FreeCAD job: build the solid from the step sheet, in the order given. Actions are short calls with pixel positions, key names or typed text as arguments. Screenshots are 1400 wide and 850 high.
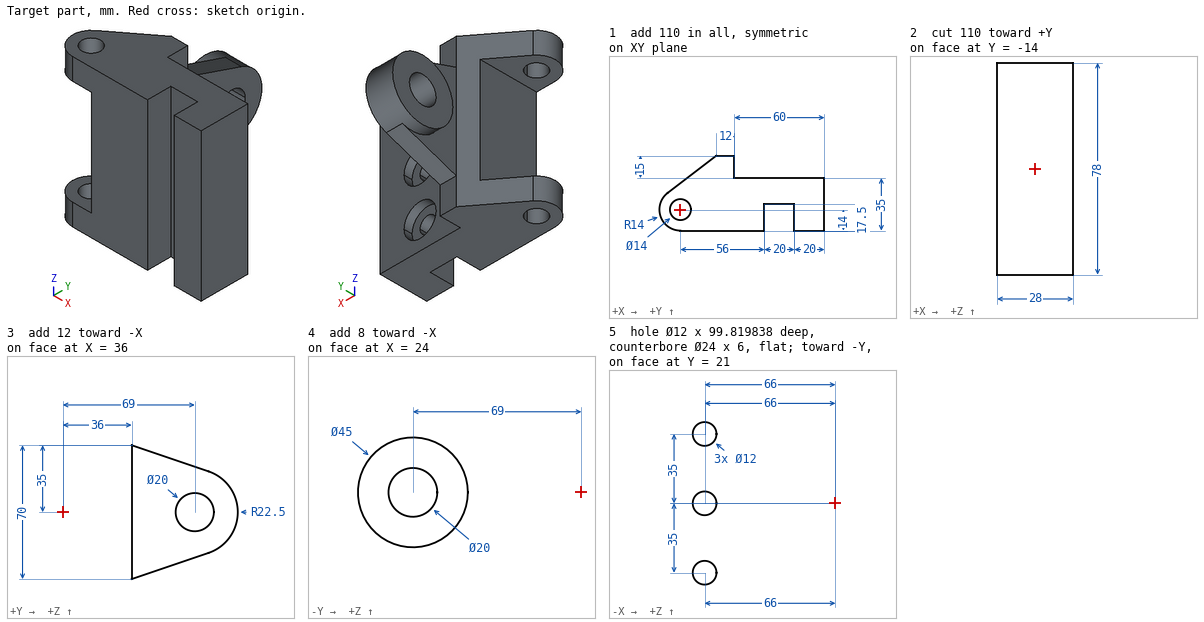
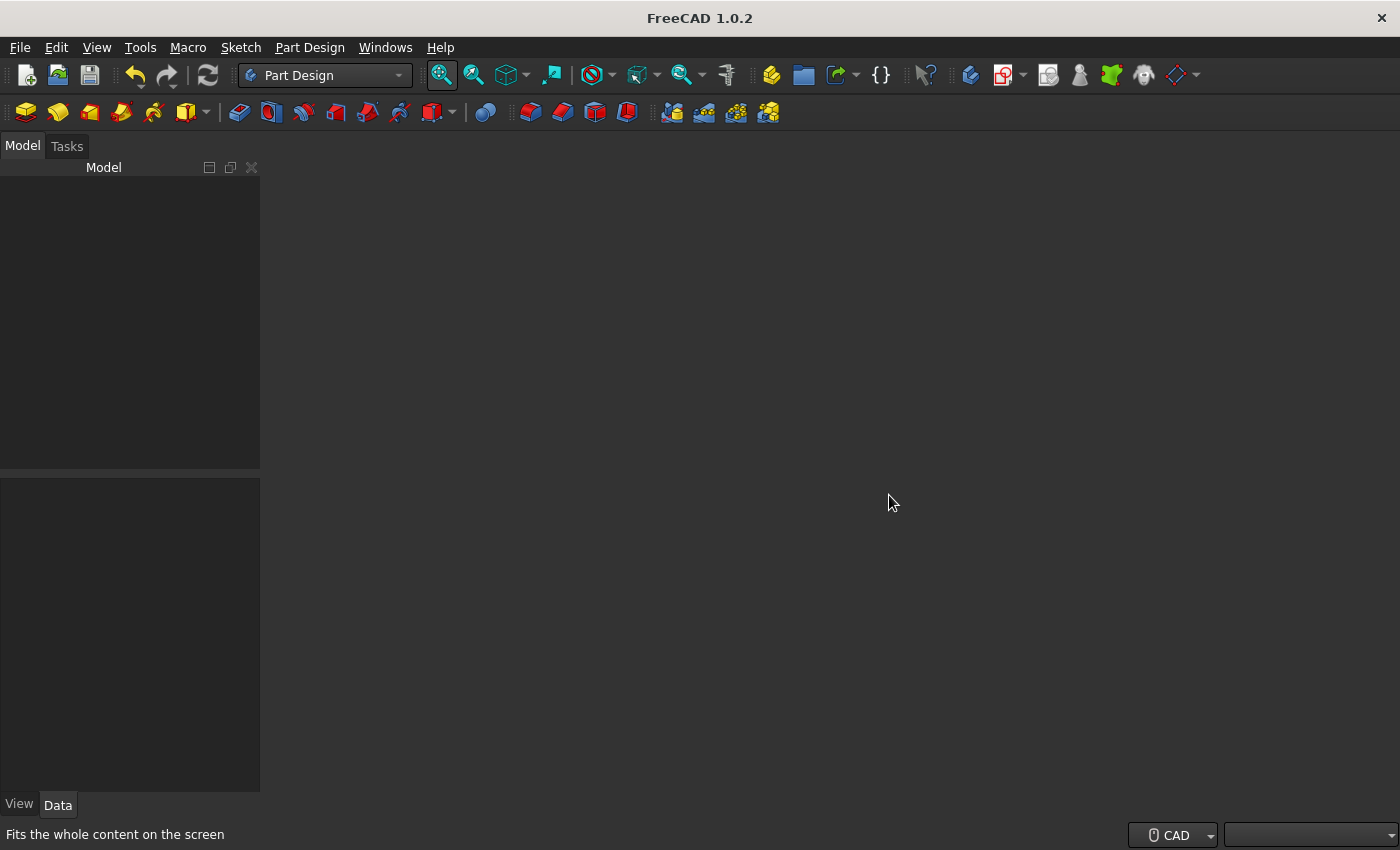
click(26, 76)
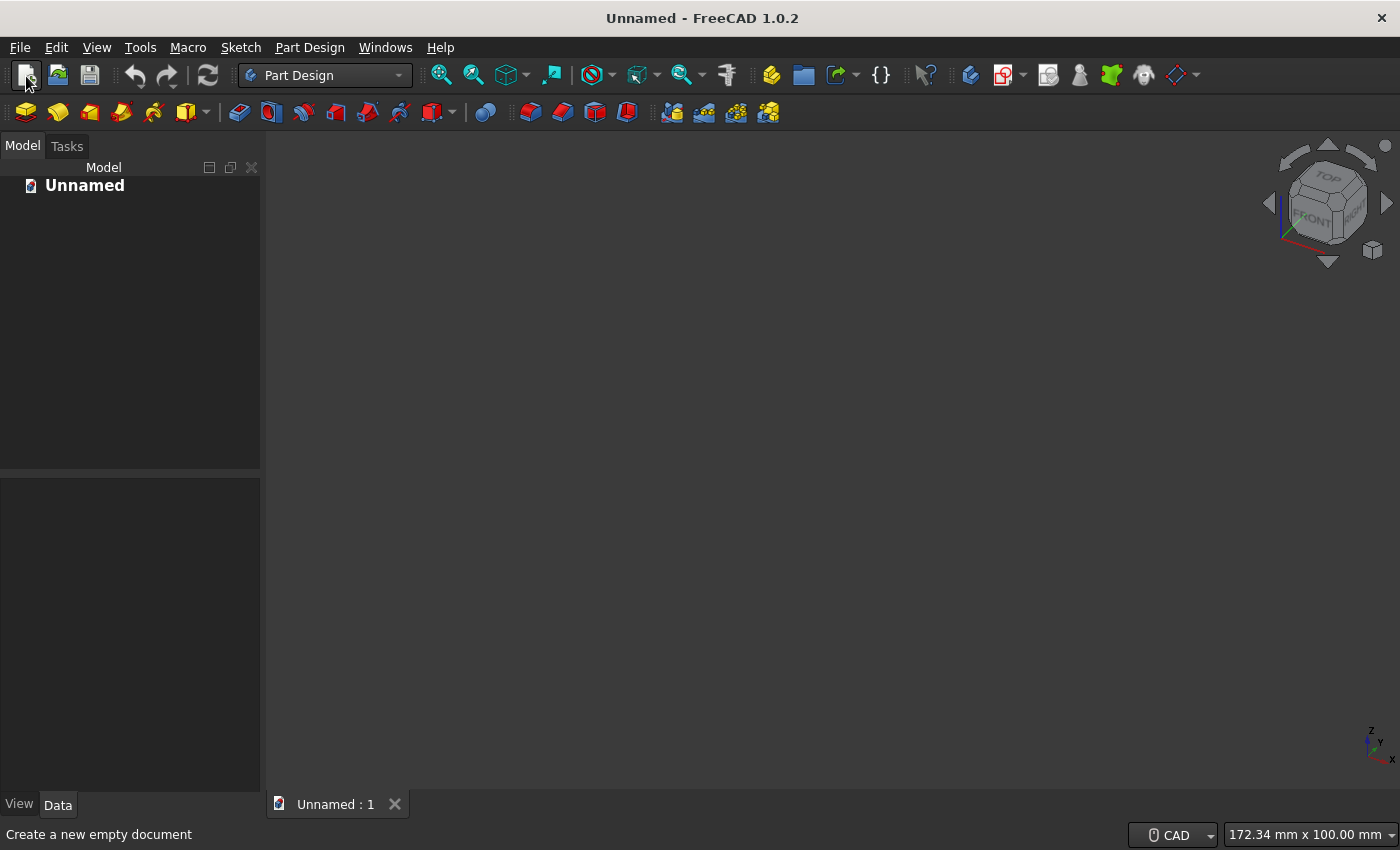
click(1004, 76)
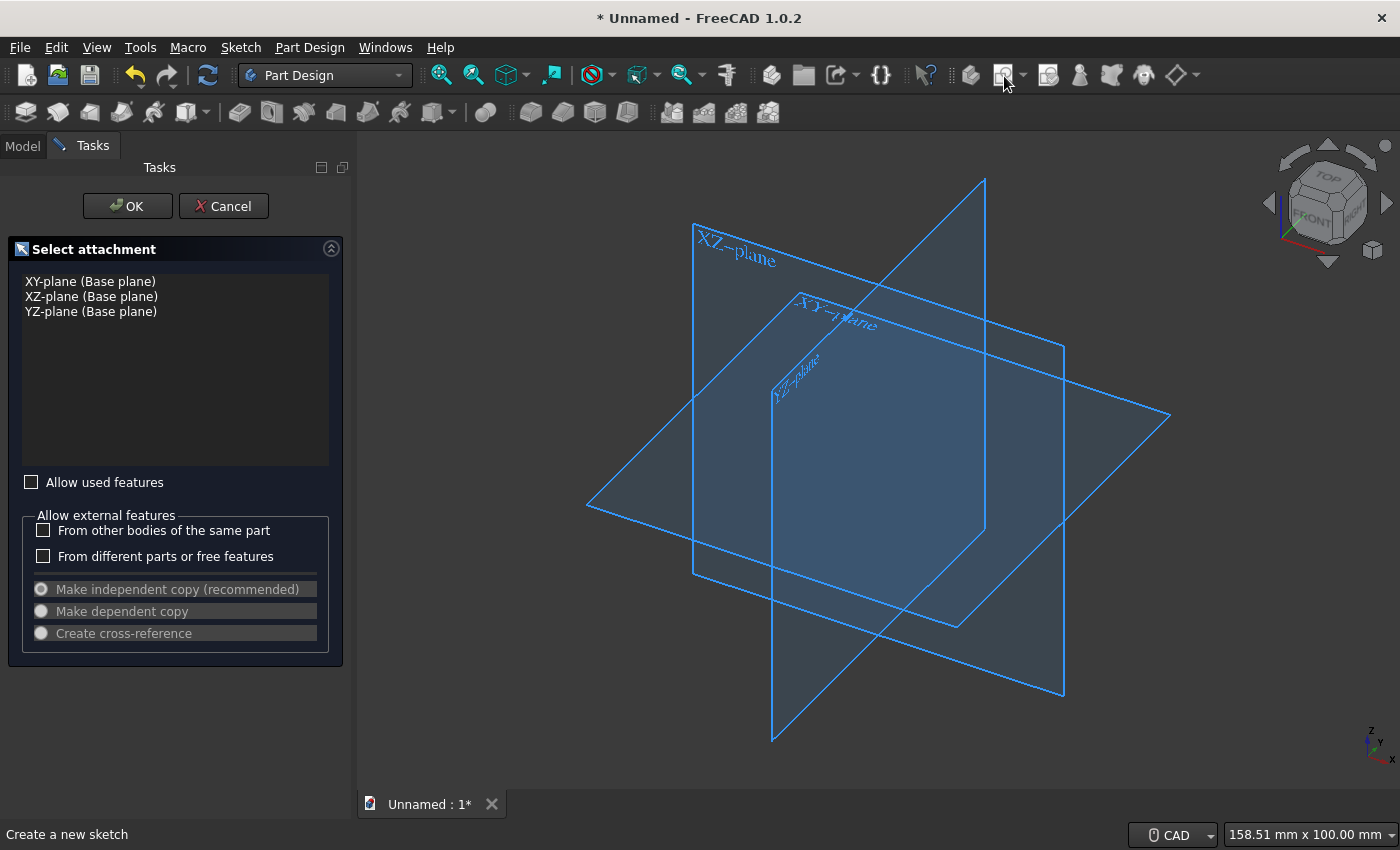
click(82, 282)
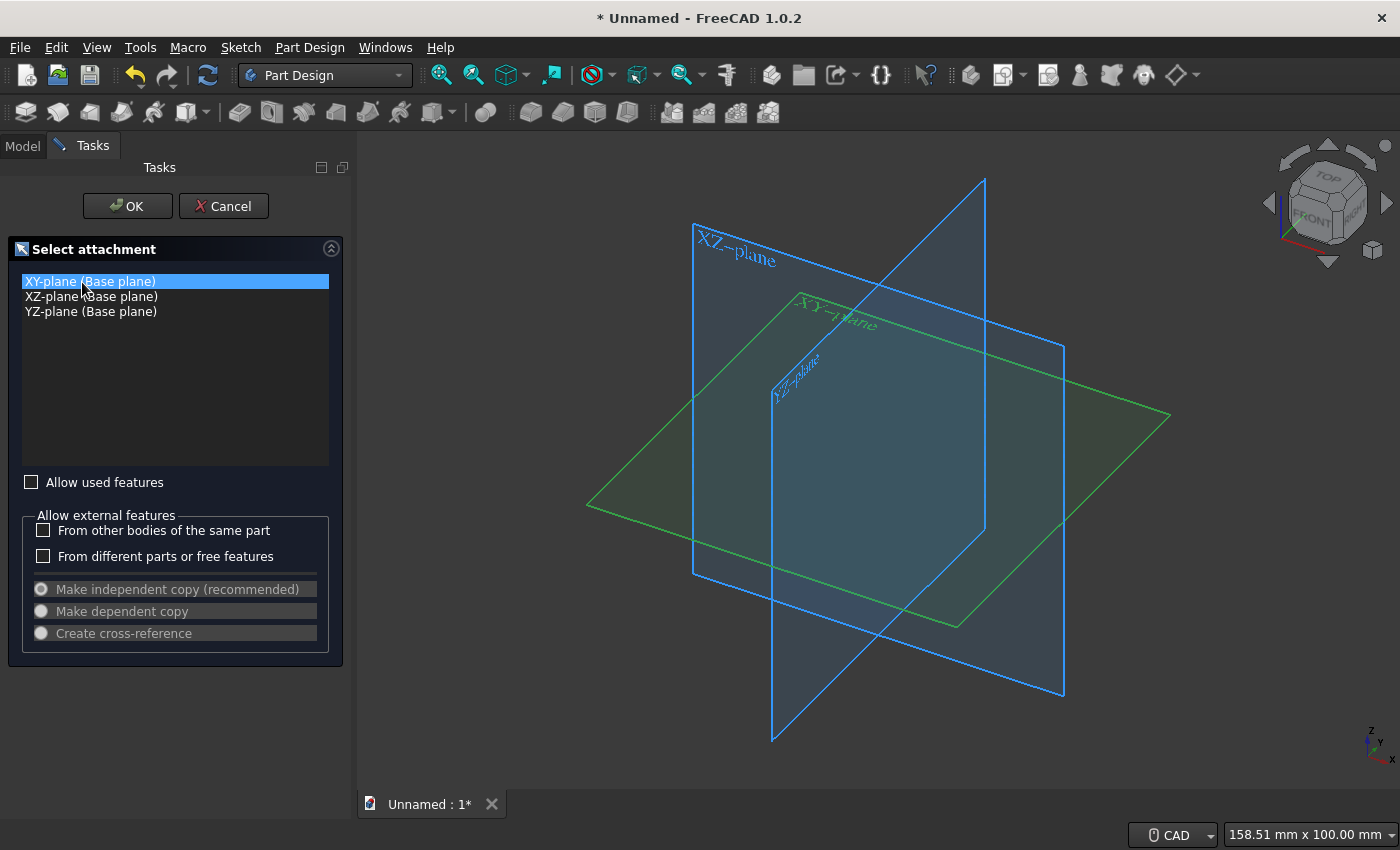
click(128, 206)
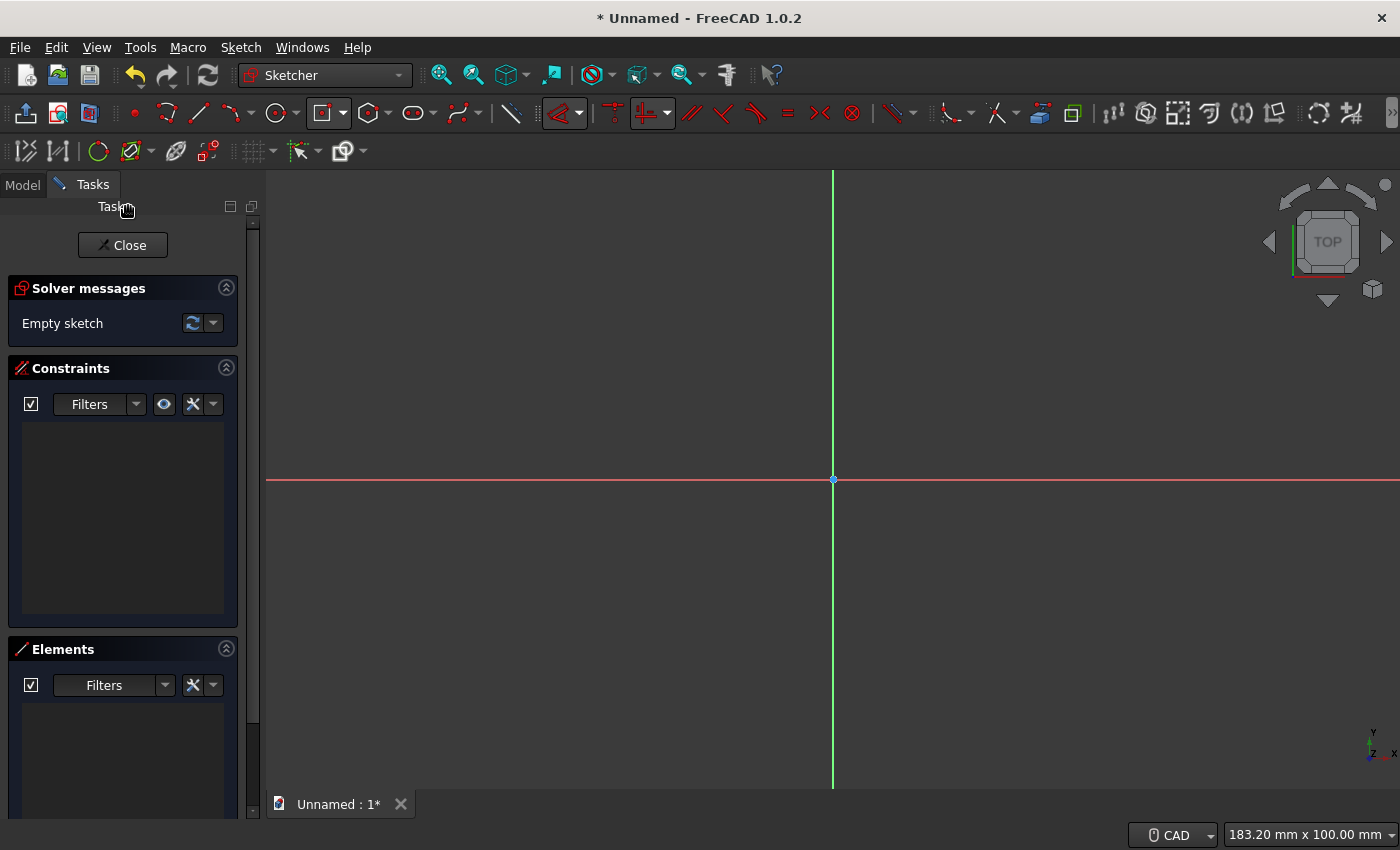
scroll(294, 618, down, 2)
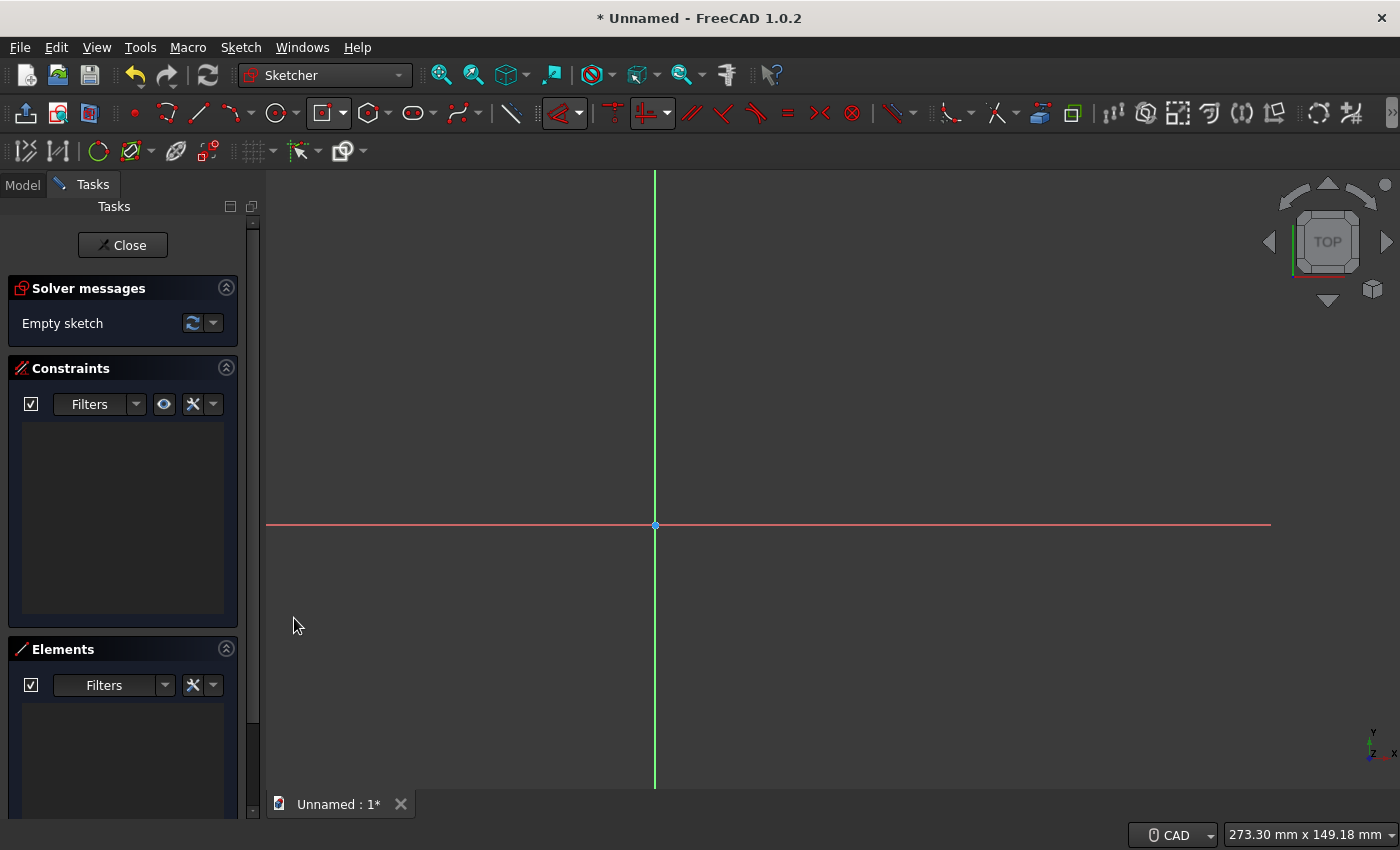
scroll(954, 480, up, 2)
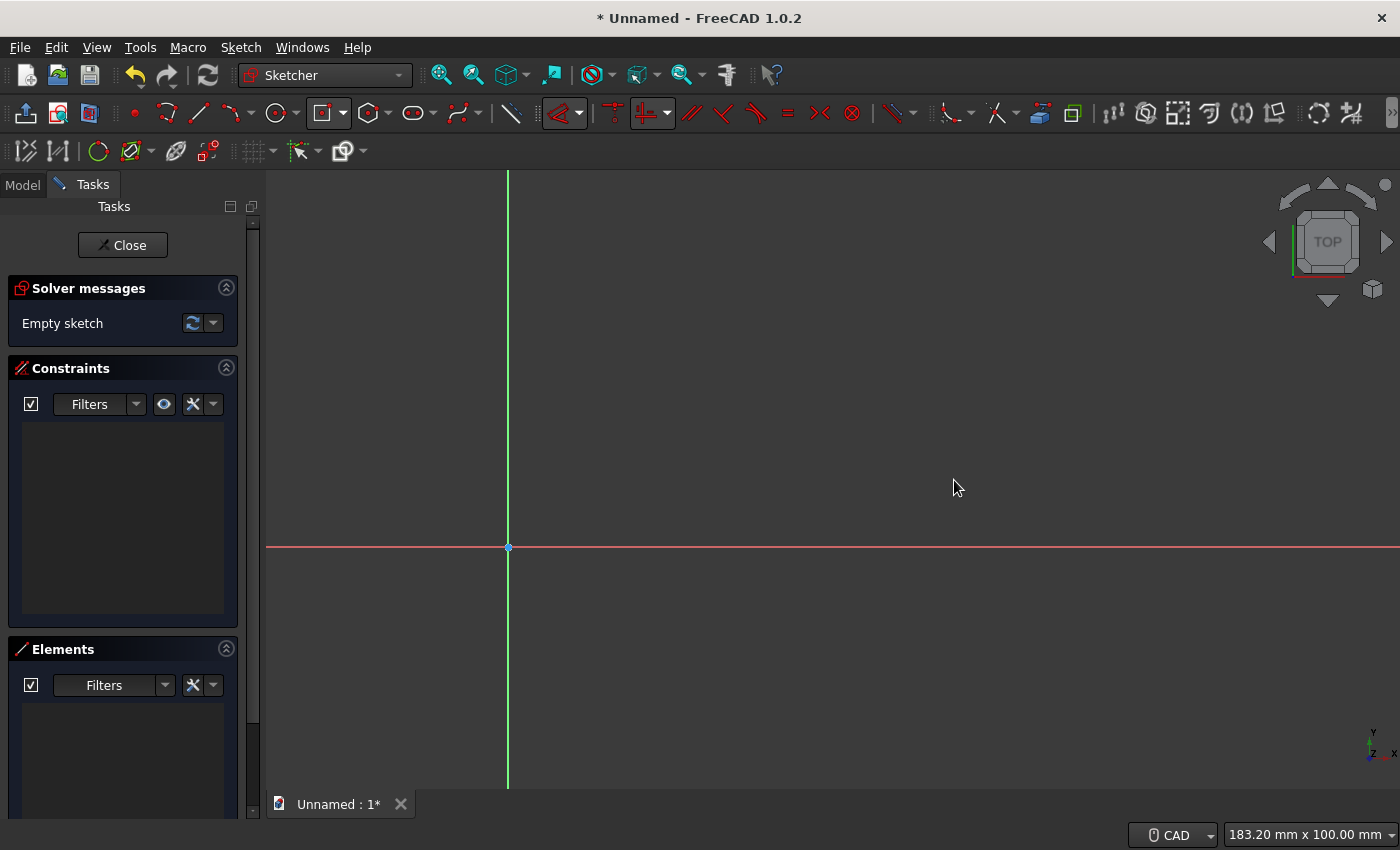
click(168, 114)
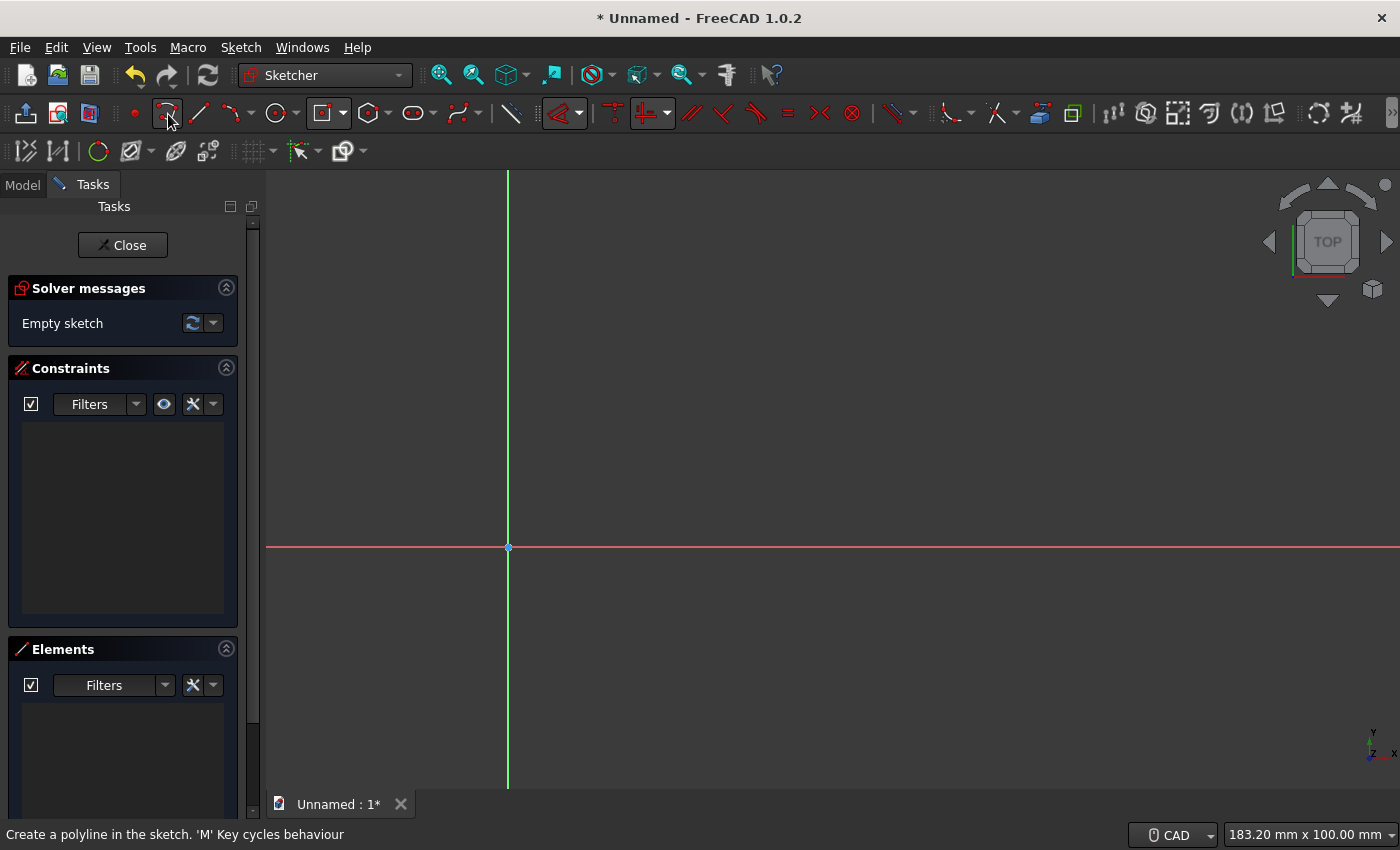
click(508, 634)
click(855, 634)
click(855, 526)
click(979, 526)
click(979, 634)
click(1102, 634)
click(1102, 417)
click(731, 417)
click(731, 325)
click(657, 325)
click(455, 479)
right_click(455, 479)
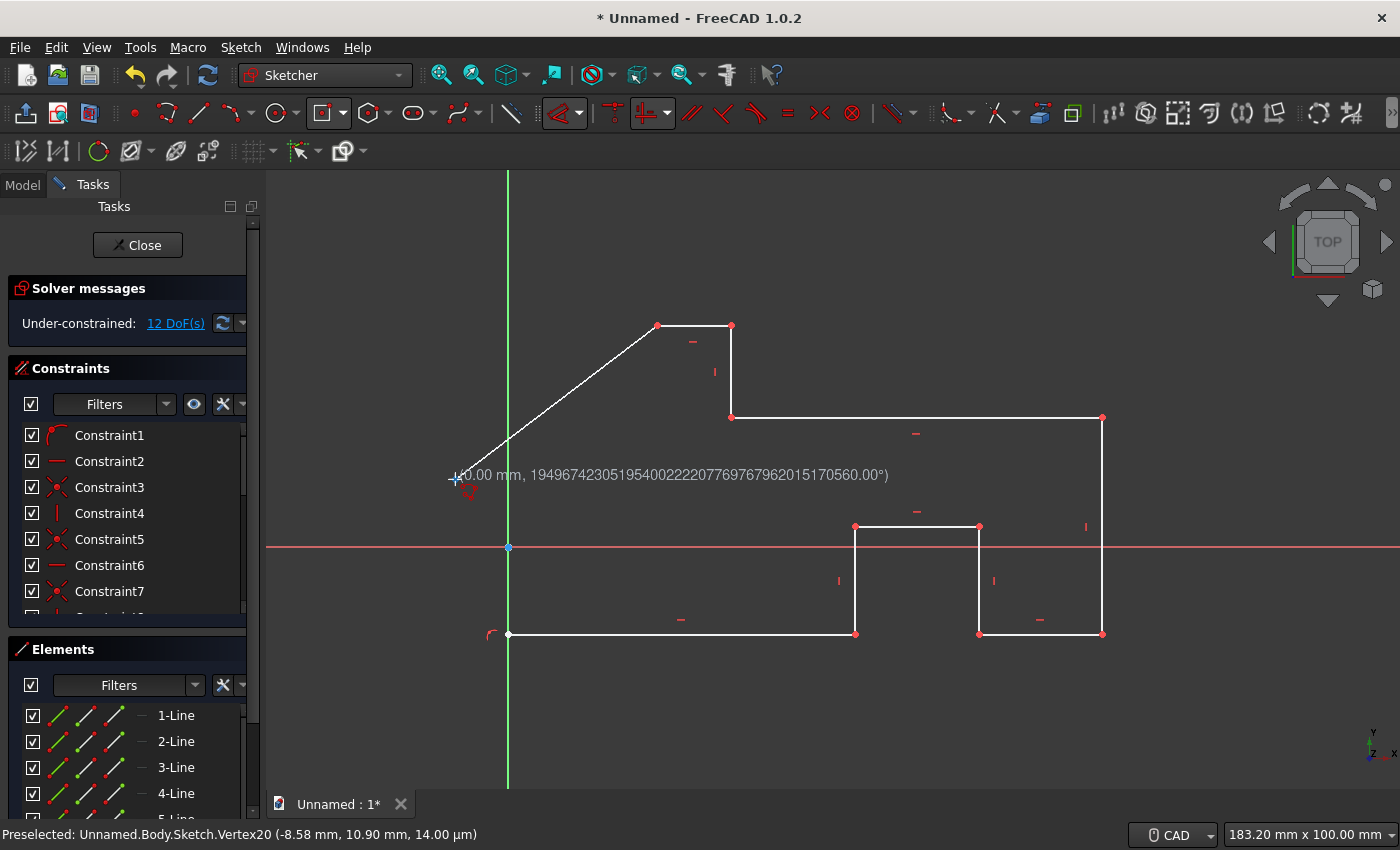
click(232, 114)